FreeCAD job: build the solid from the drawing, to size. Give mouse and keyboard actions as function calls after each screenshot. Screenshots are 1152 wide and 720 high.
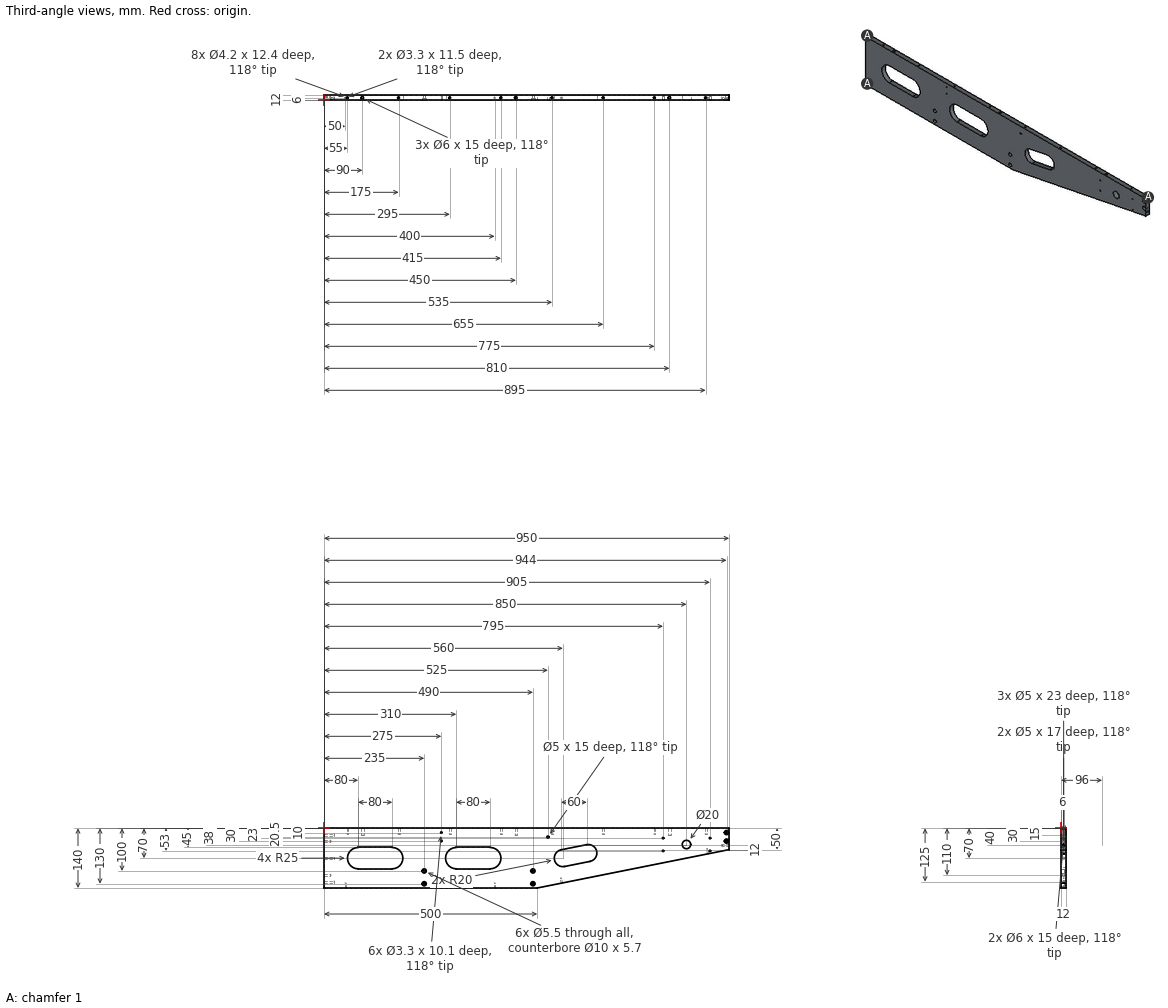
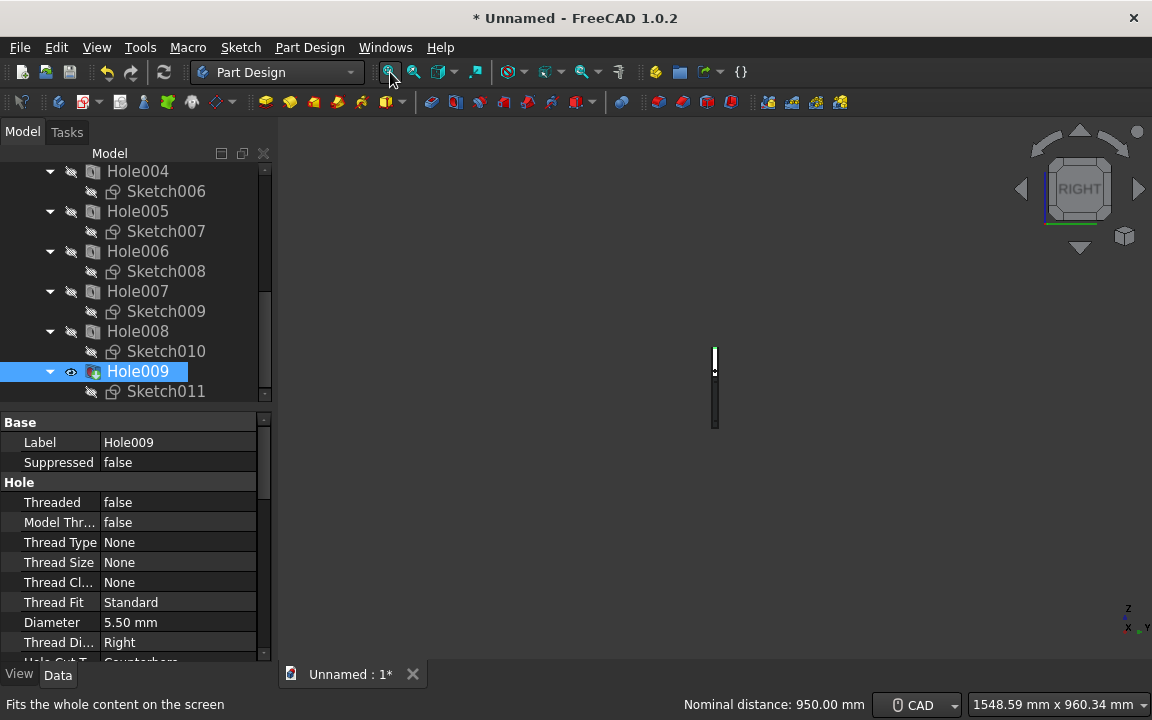
key(5)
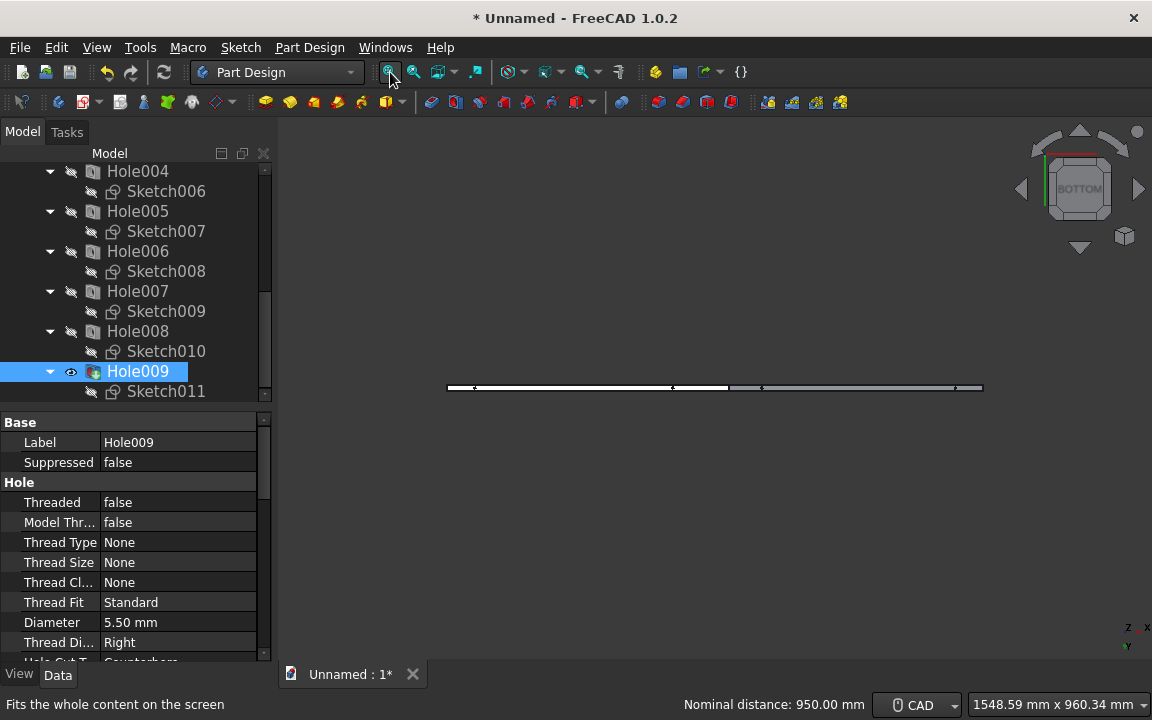
scroll(447, 387, up, 9)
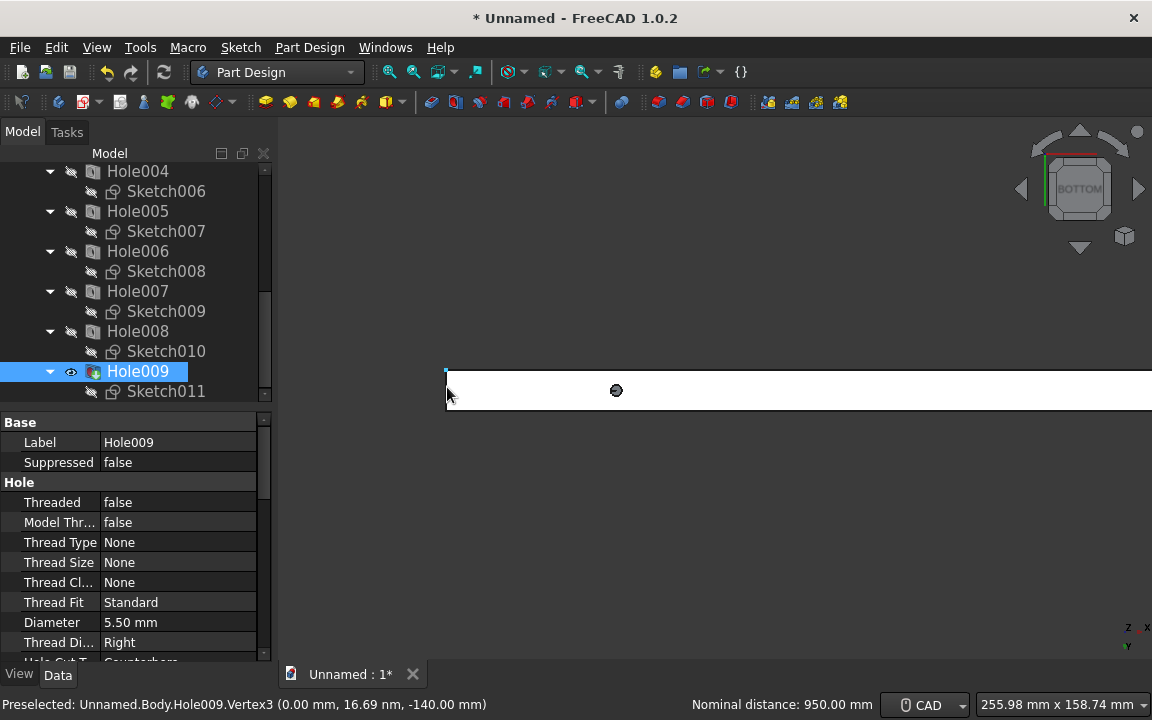
click(446, 390, ctrl)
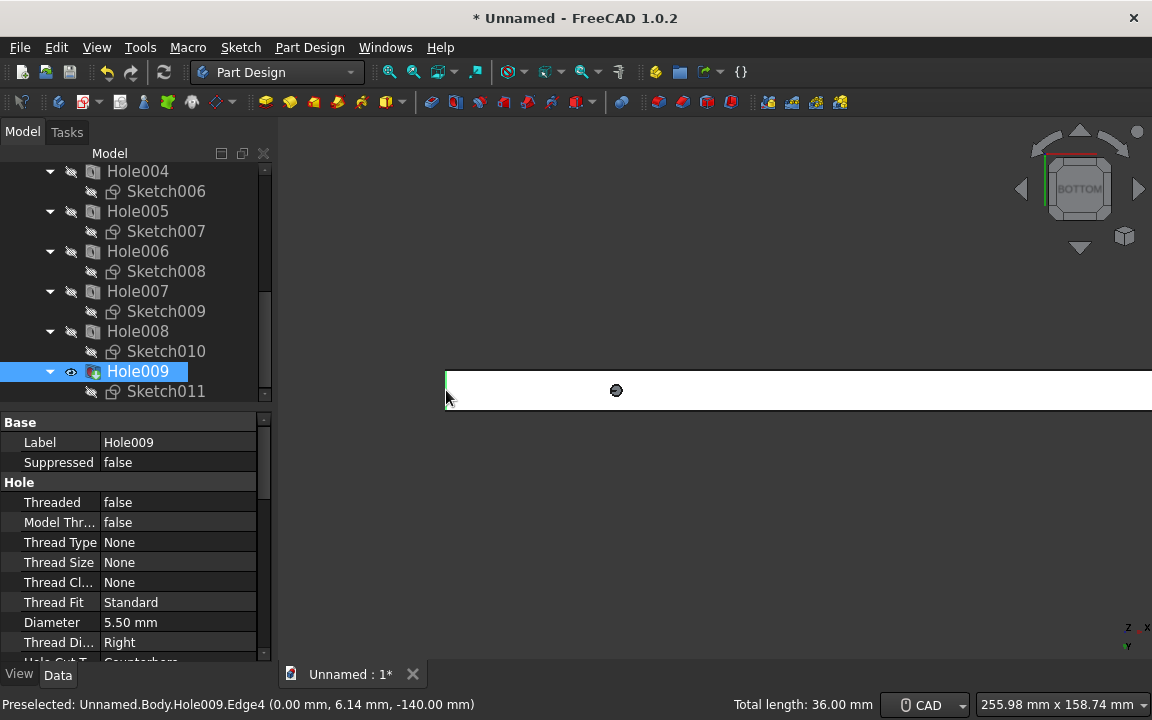
click(684, 102)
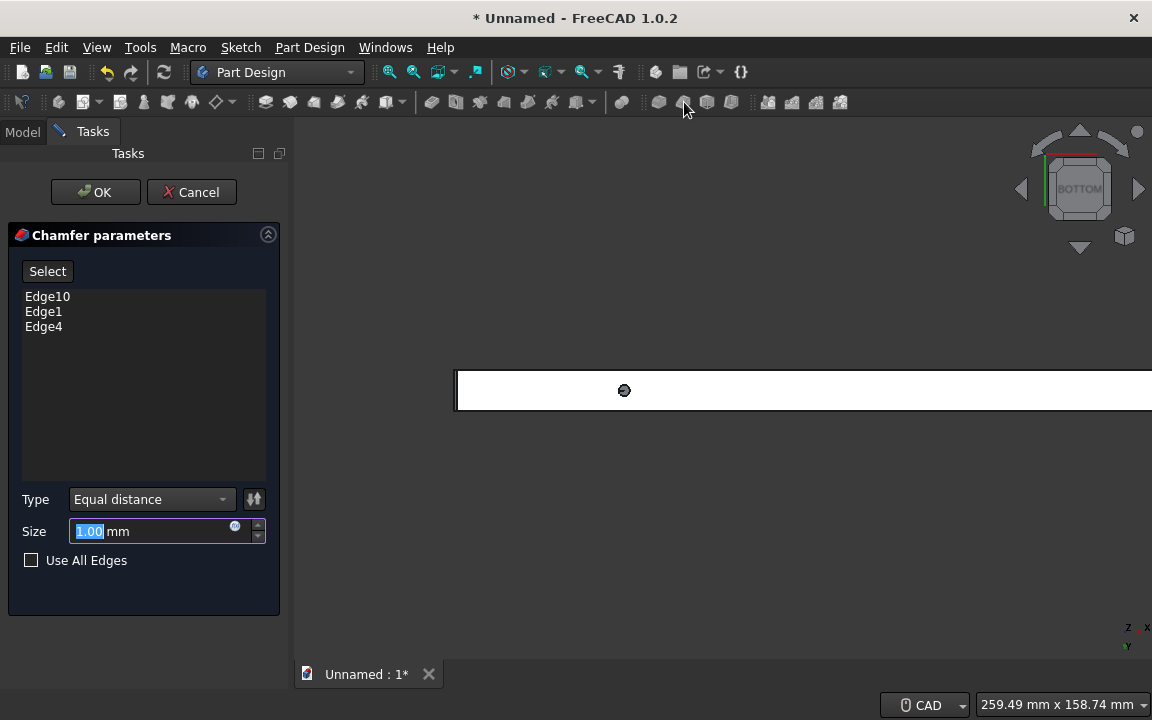
text(1)
key(Tab)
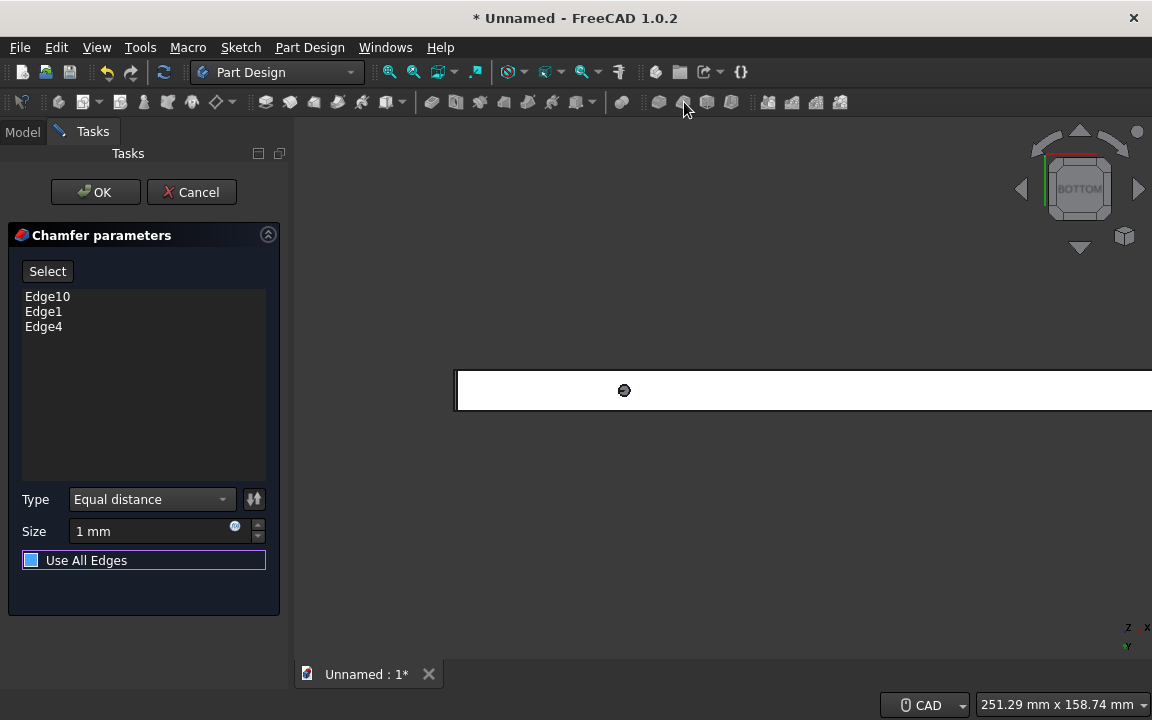
click(96, 192)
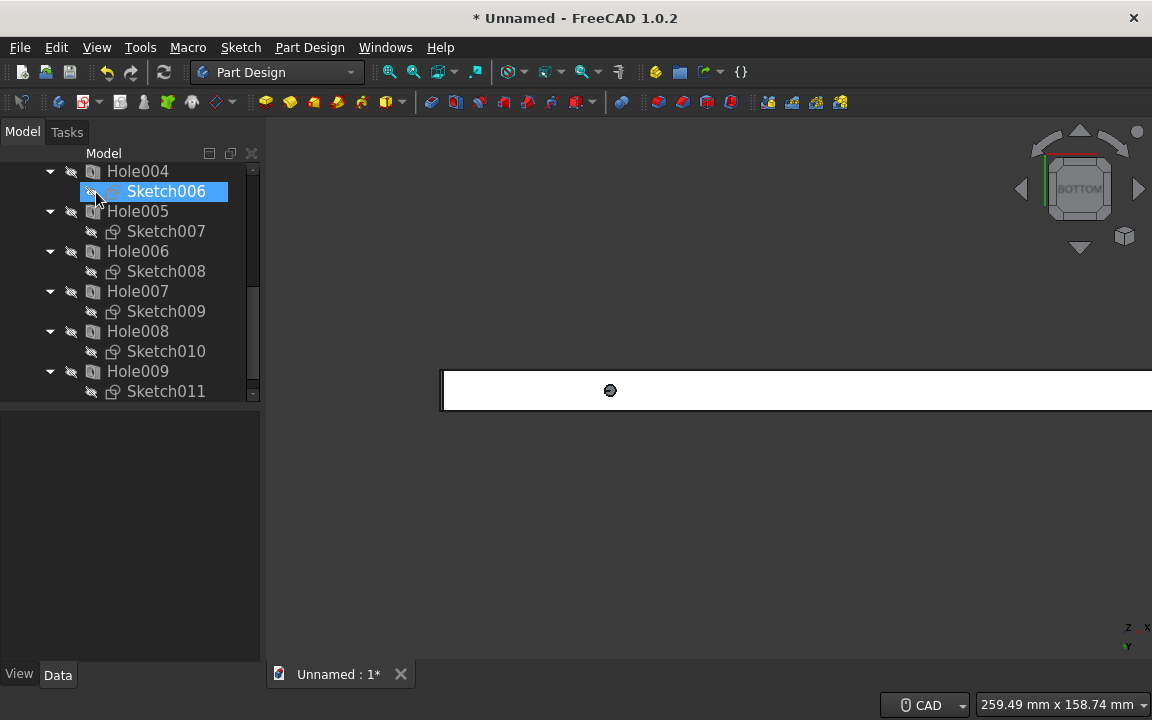
key(0)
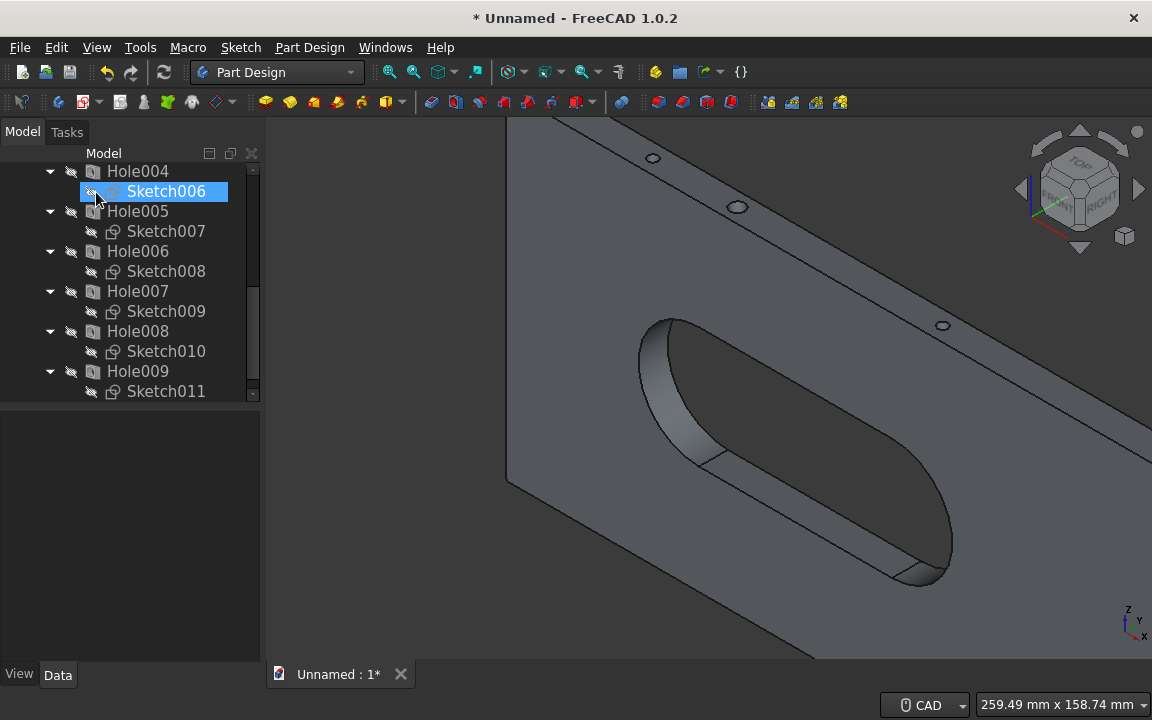
key(v)
key(f)